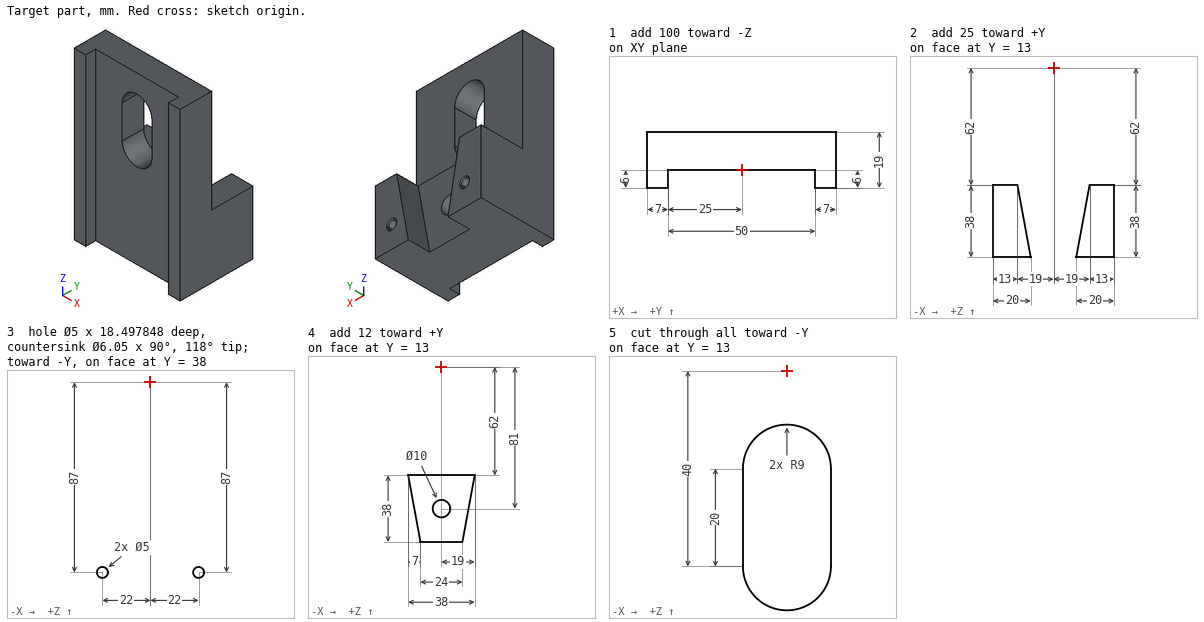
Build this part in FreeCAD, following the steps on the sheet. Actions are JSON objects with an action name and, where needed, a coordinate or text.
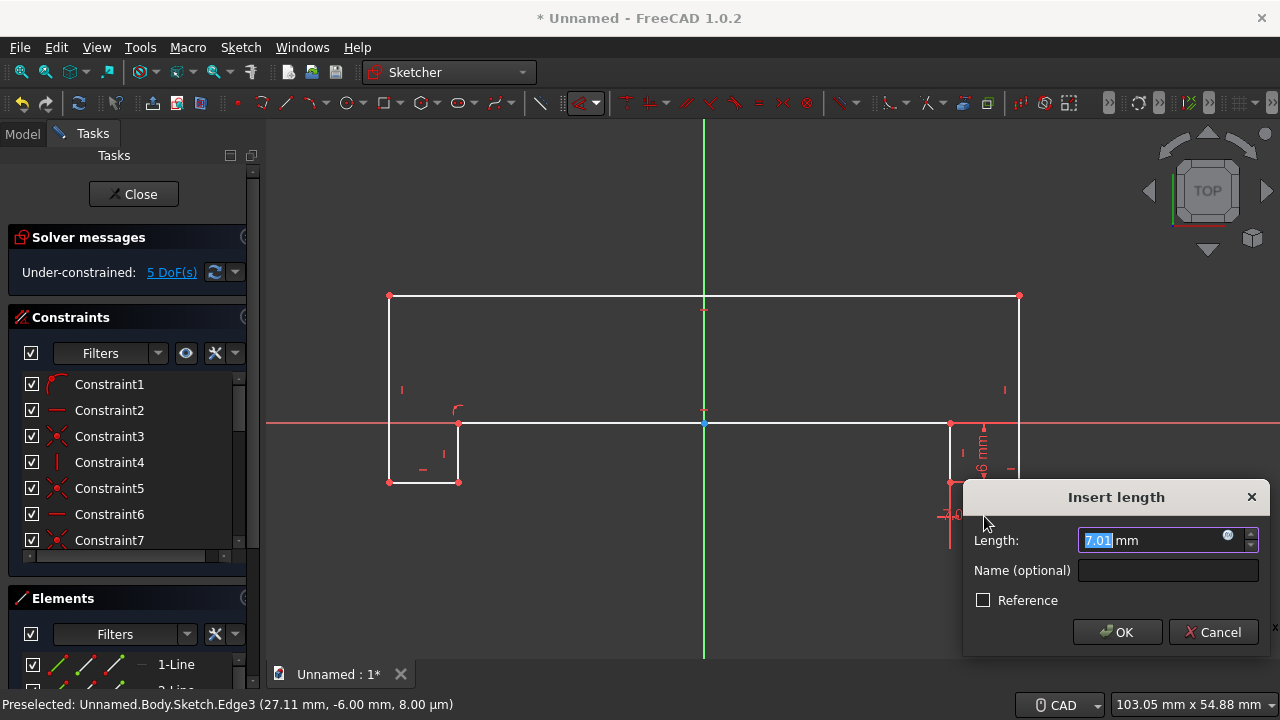
{"action": "type", "text": "7"}
{"action": "key", "text": "Return"}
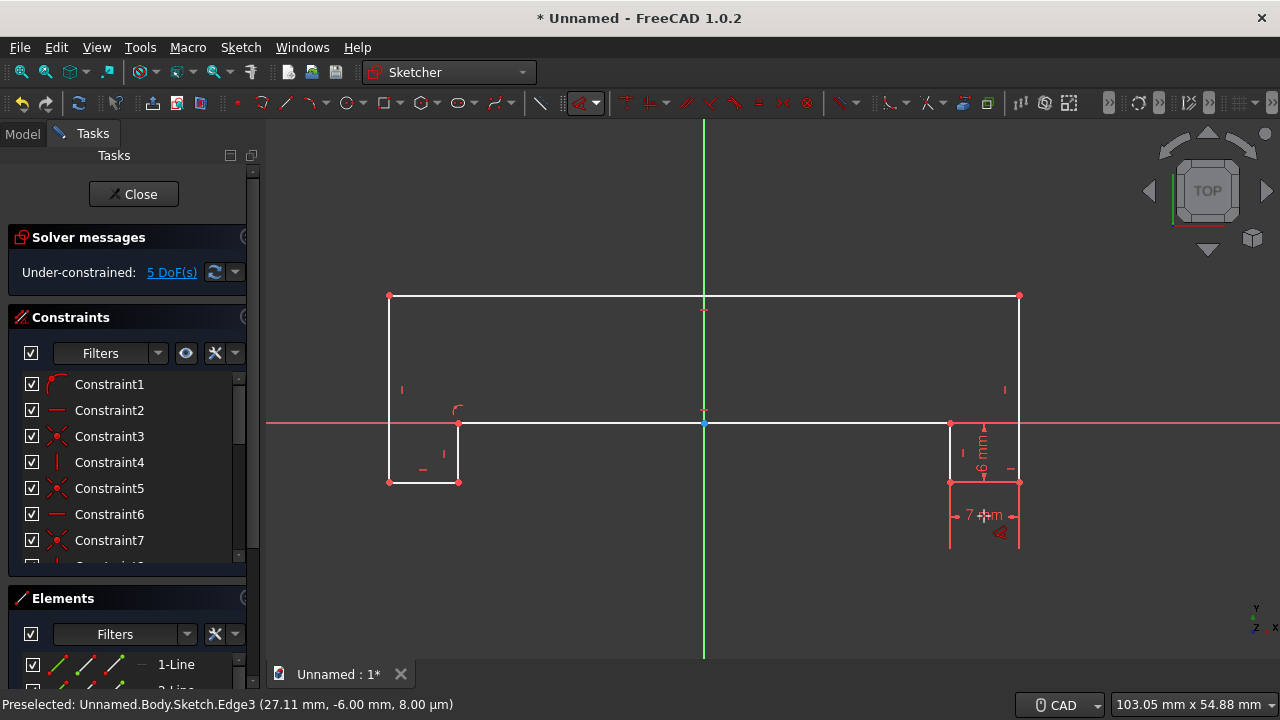
{"action": "left_click", "coordinate": [410, 483]}
{"action": "left_click", "coordinate": [424, 517]}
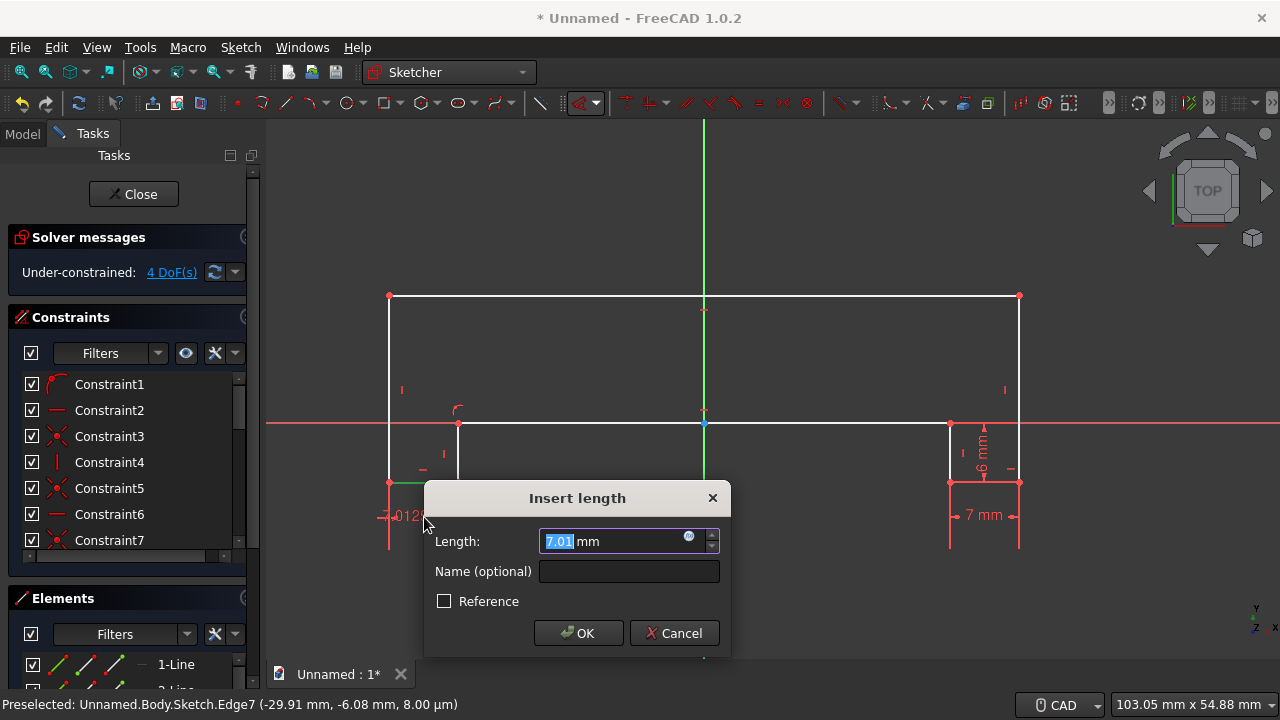
{"action": "type", "text": "7"}
{"action": "key", "text": "Return"}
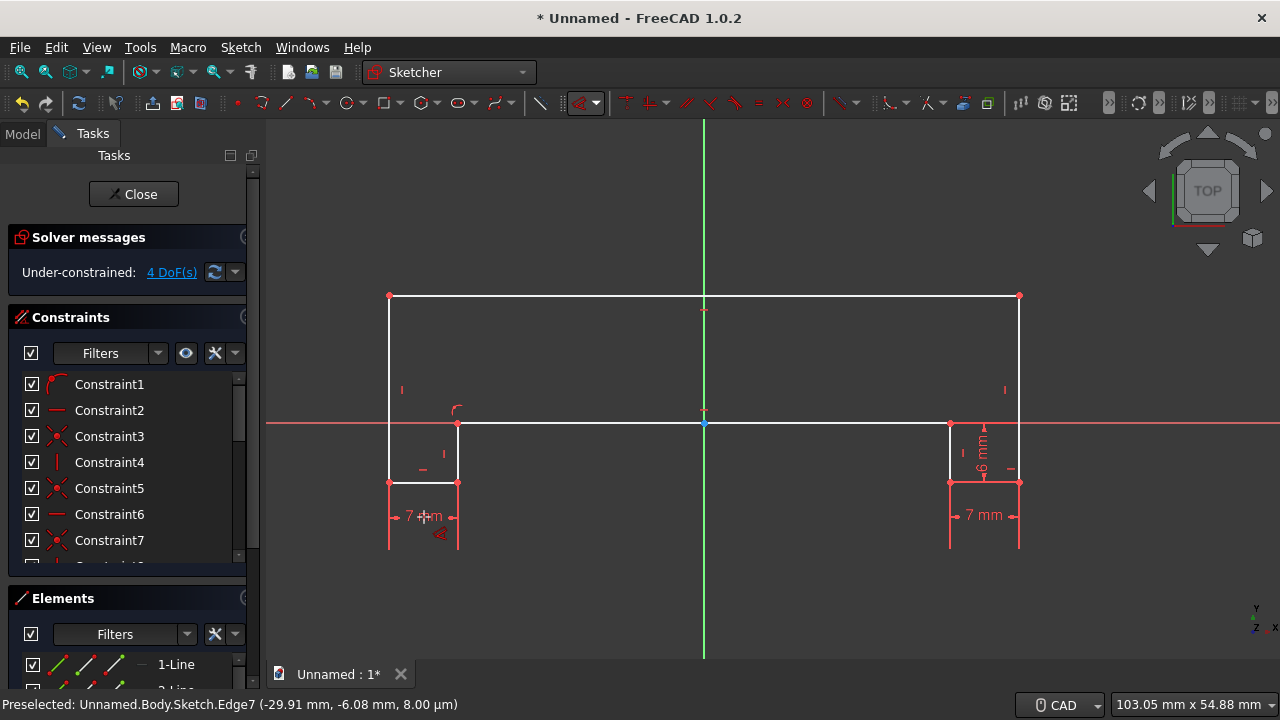
{"action": "left_click", "coordinate": [458, 465]}
{"action": "left_click", "coordinate": [424, 453]}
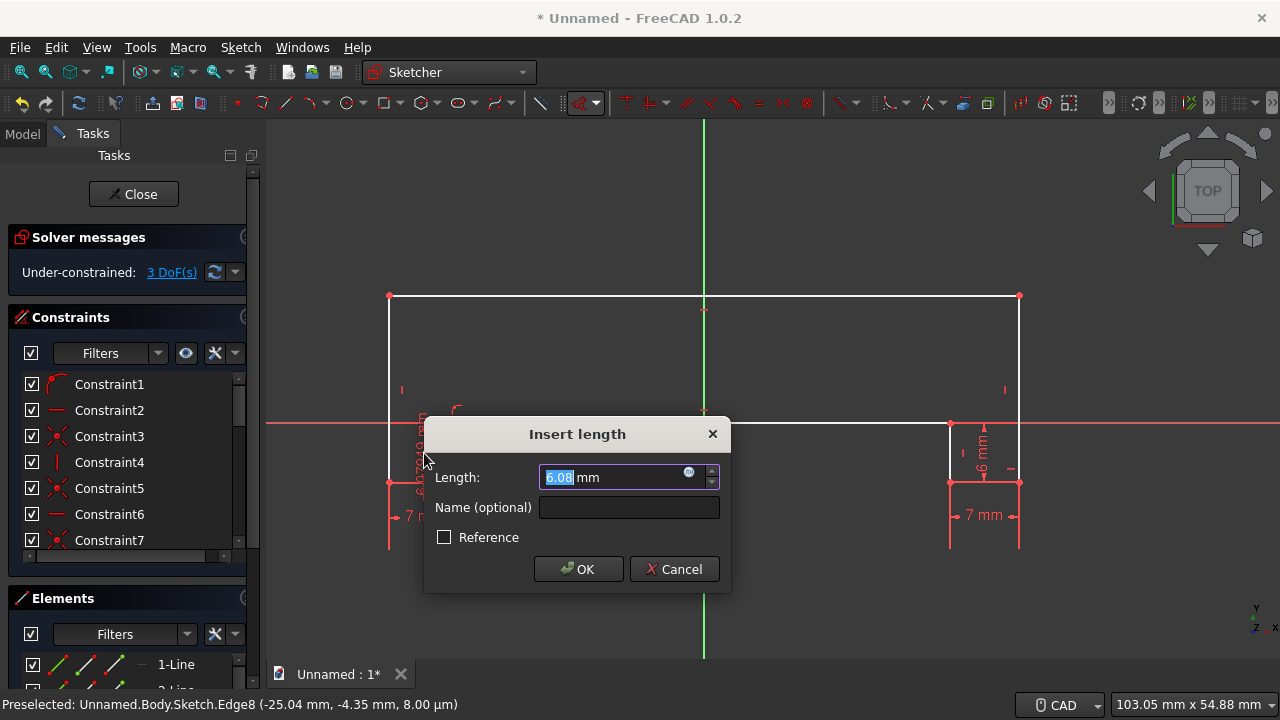
{"action": "type", "text": "6"}
{"action": "key", "text": "Return"}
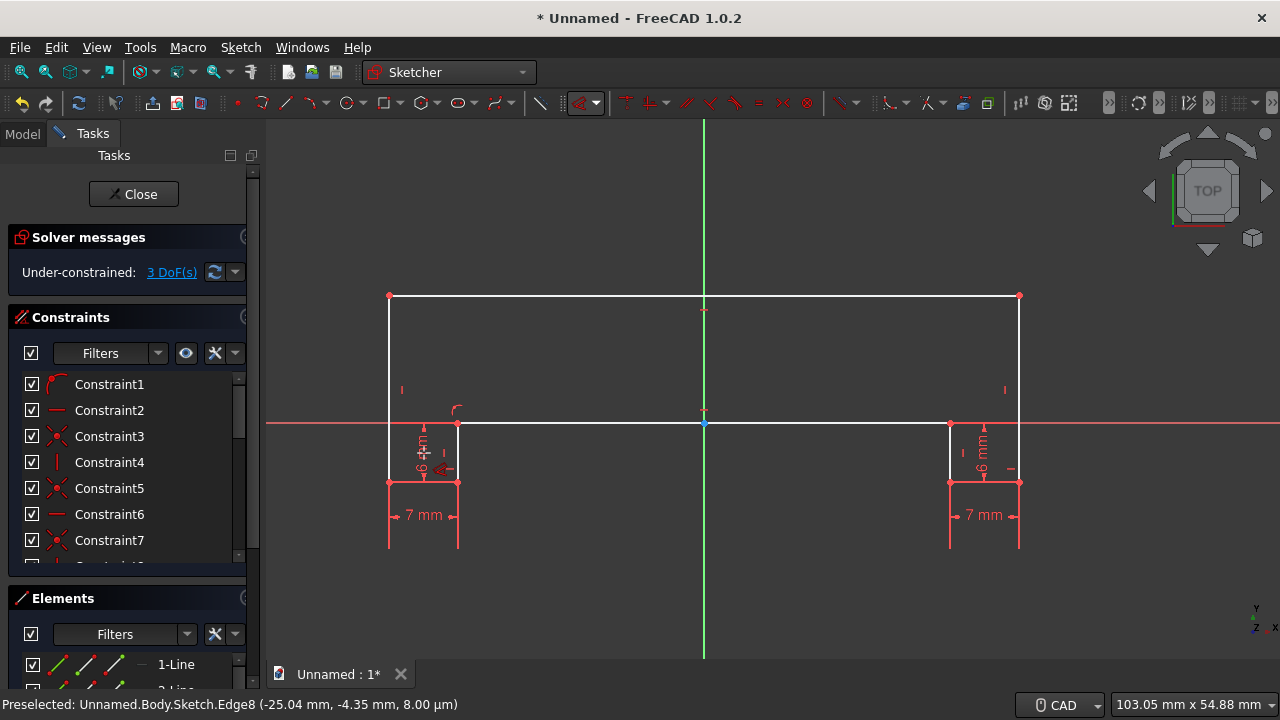
{"action": "left_click", "coordinate": [606, 423]}
{"action": "left_click", "coordinate": [591, 457]}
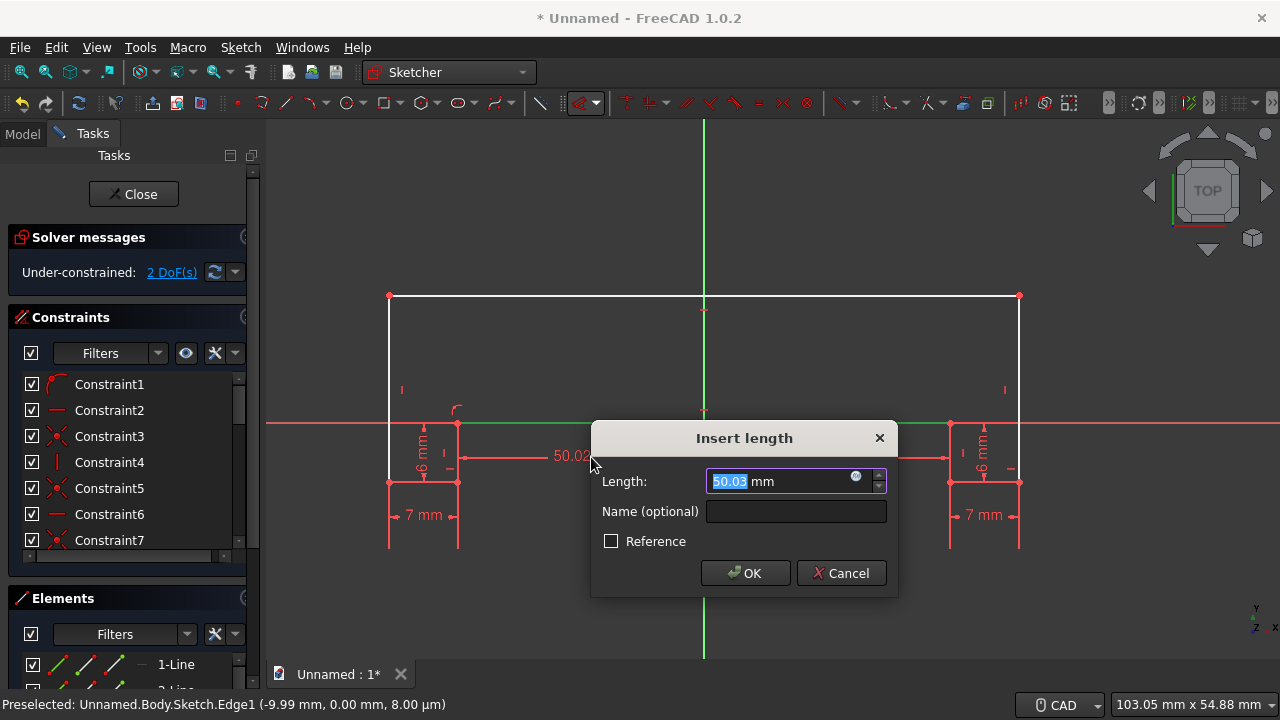
{"action": "type", "text": "50"}
{"action": "key", "text": "Return"}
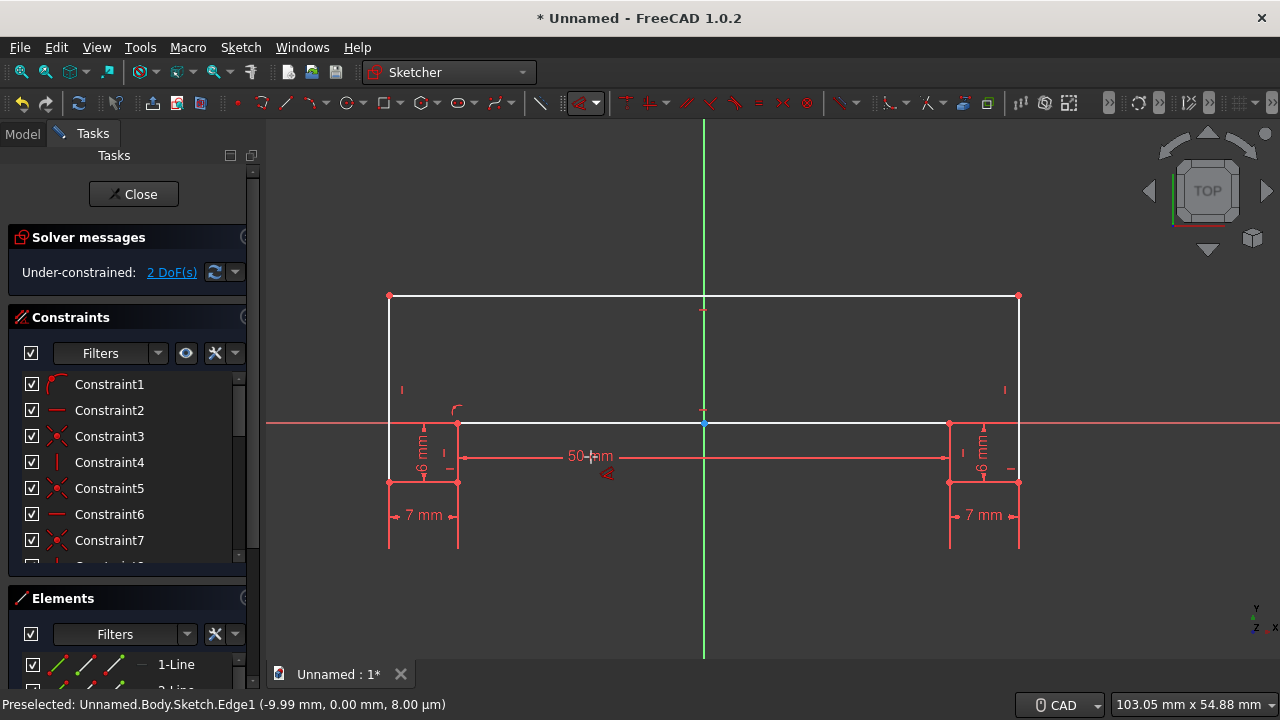
{"action": "left_click", "coordinate": [1019, 426]}
{"action": "left_click", "coordinate": [1053, 389]}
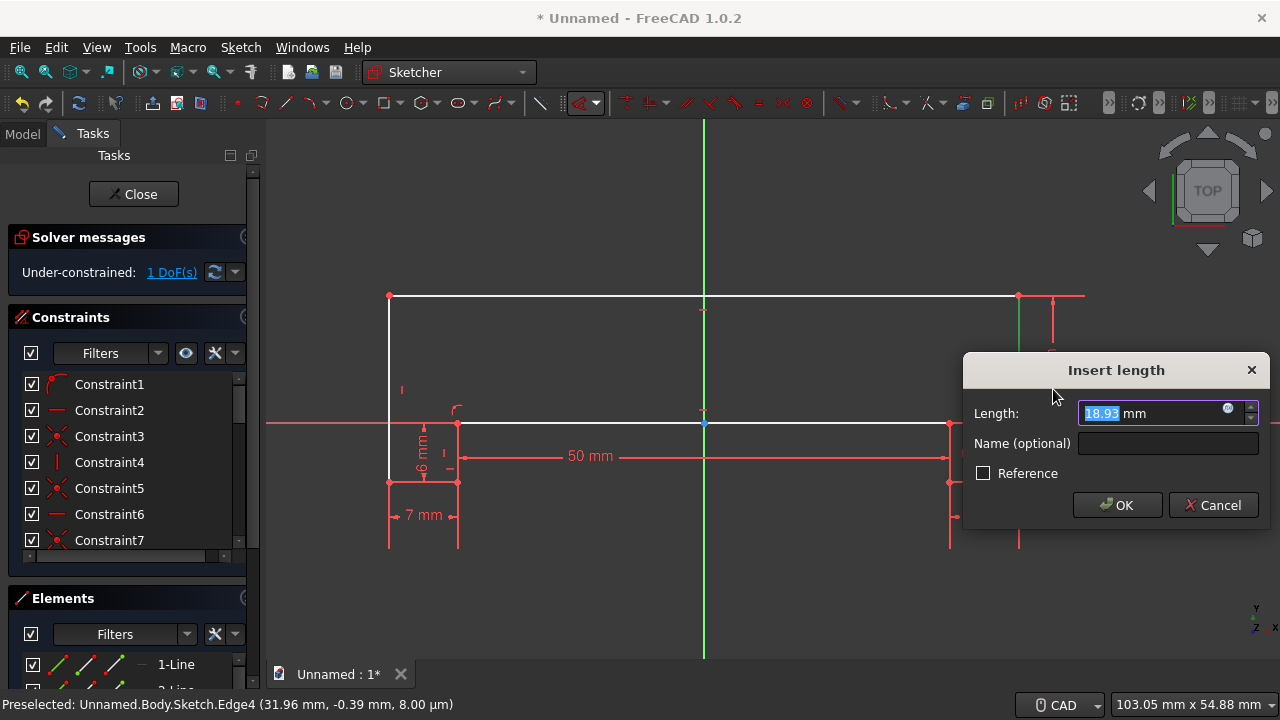
{"action": "type", "text": "19"}
{"action": "key", "text": "Return"}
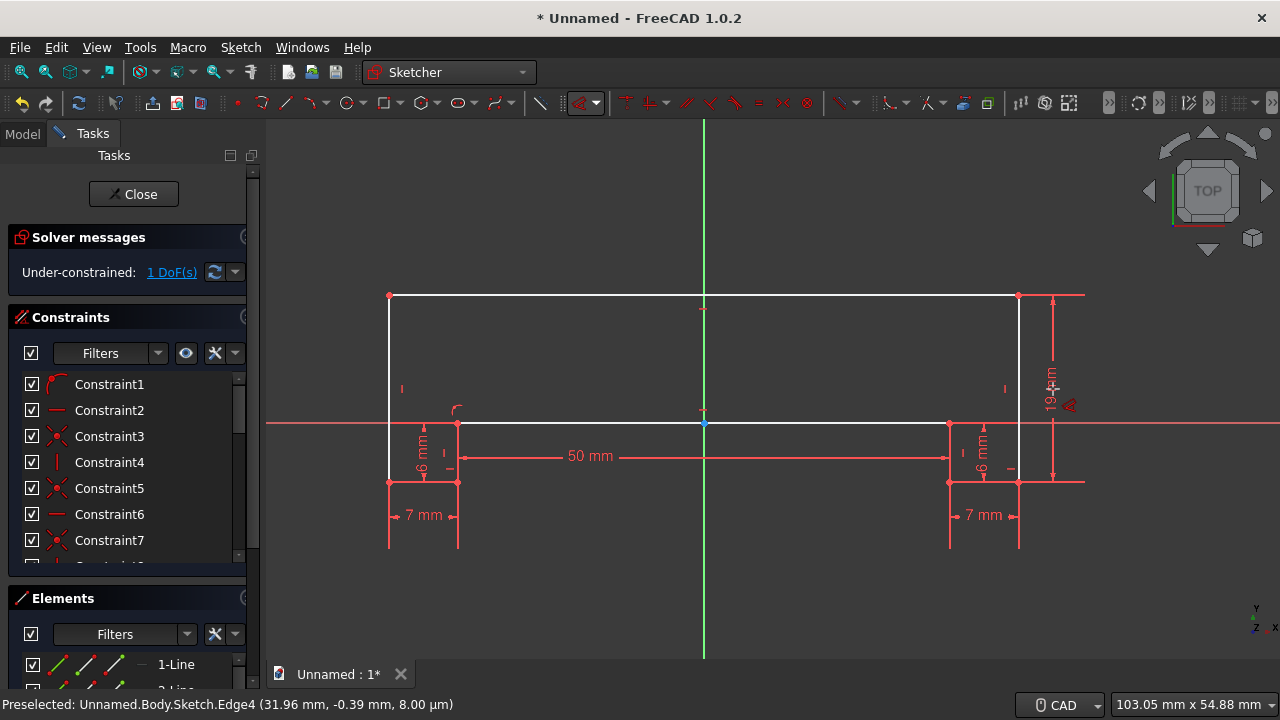
{"action": "left_click", "coordinate": [458, 423]}
{"action": "left_click", "coordinate": [495, 457]}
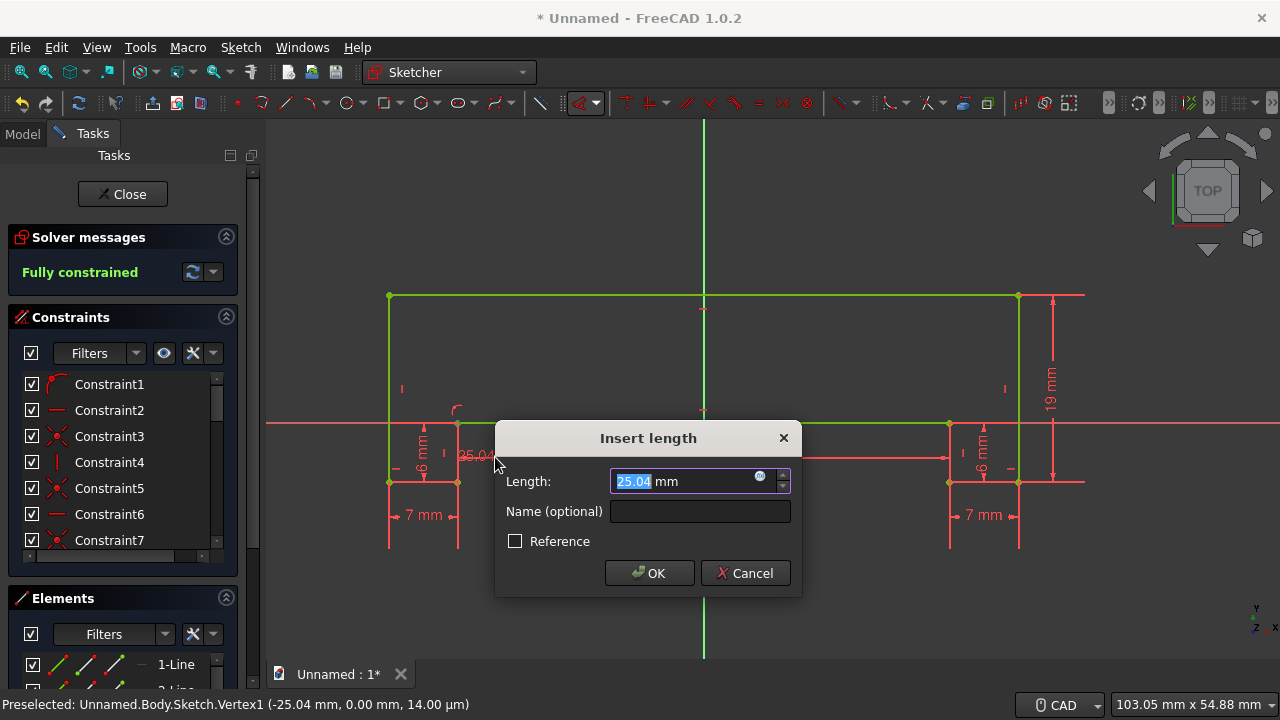
{"action": "type", "text": "25"}
{"action": "key", "text": "Return"}
{"action": "key", "text": "Escape"}